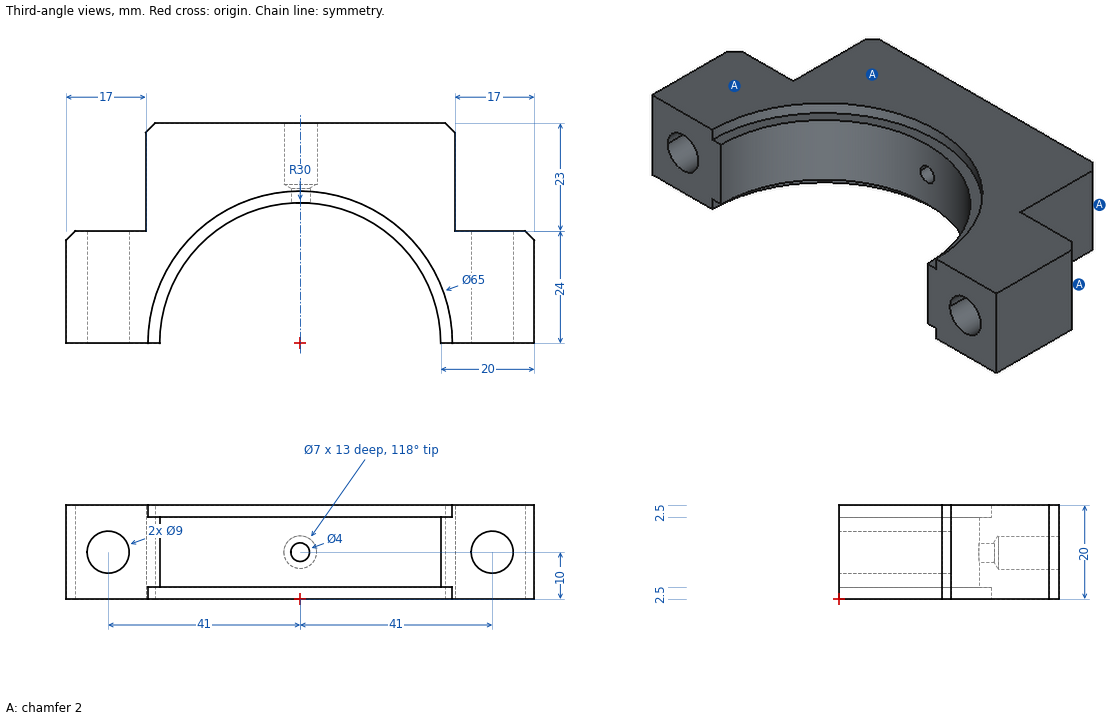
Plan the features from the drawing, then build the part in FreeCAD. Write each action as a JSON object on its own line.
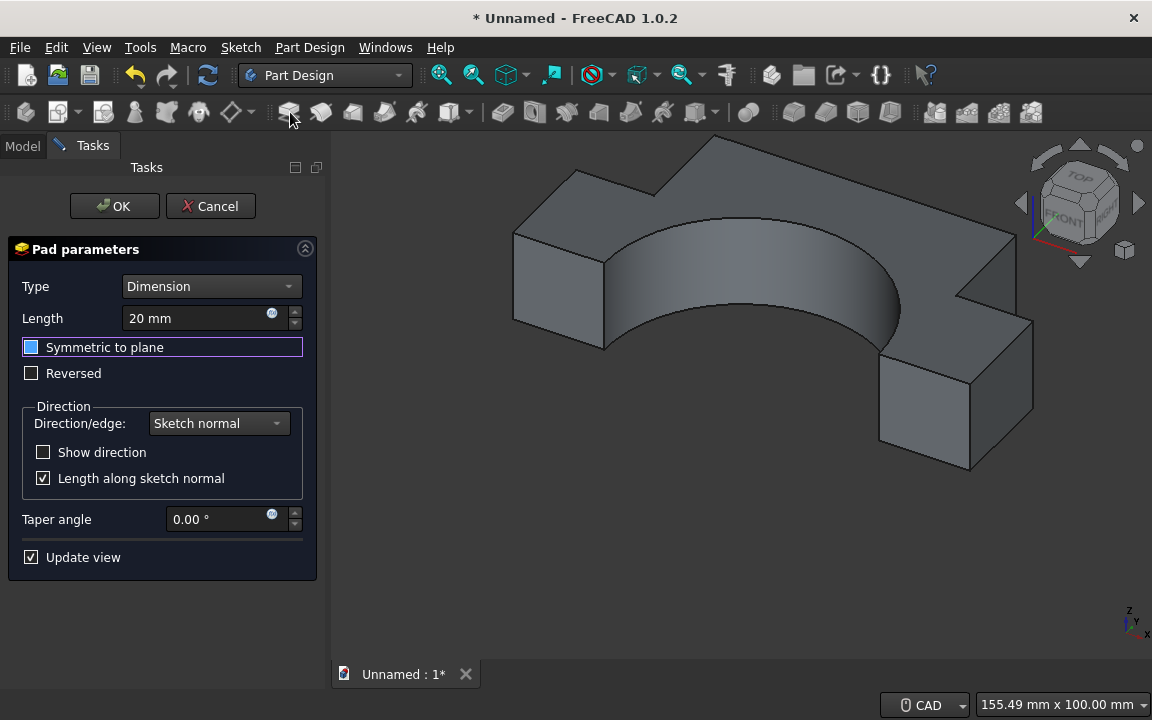
{"action": "left_click", "coordinate": [115, 206]}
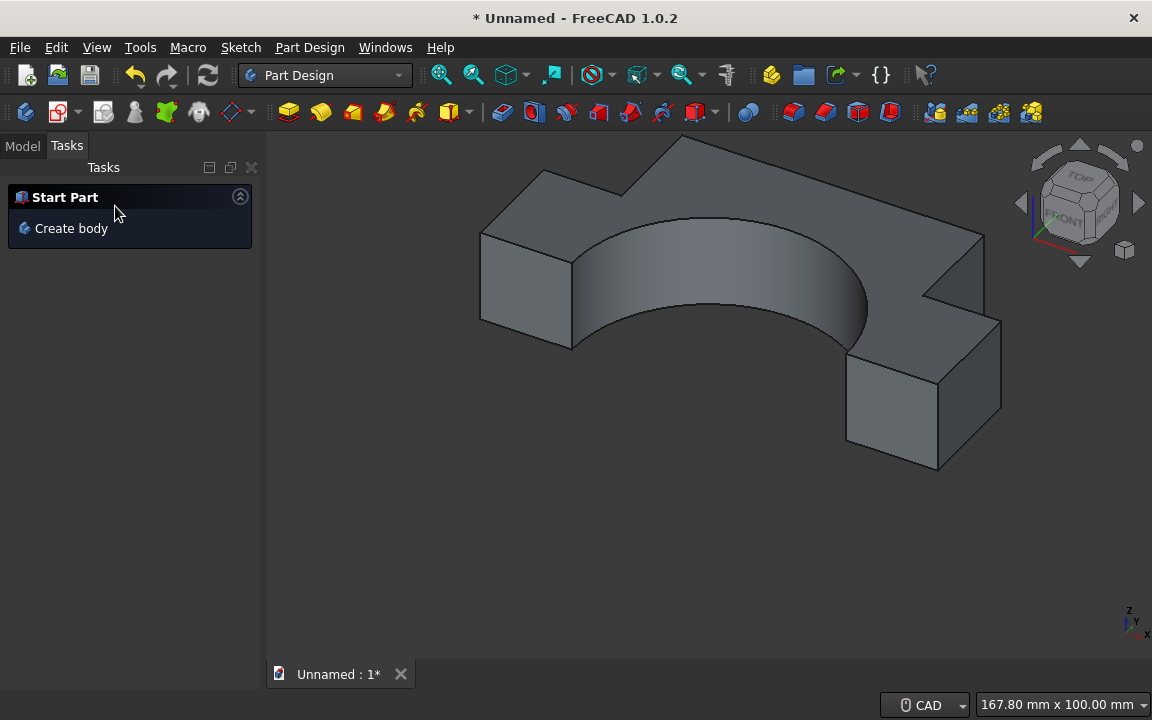
{"action": "left_click", "coordinate": [442, 76]}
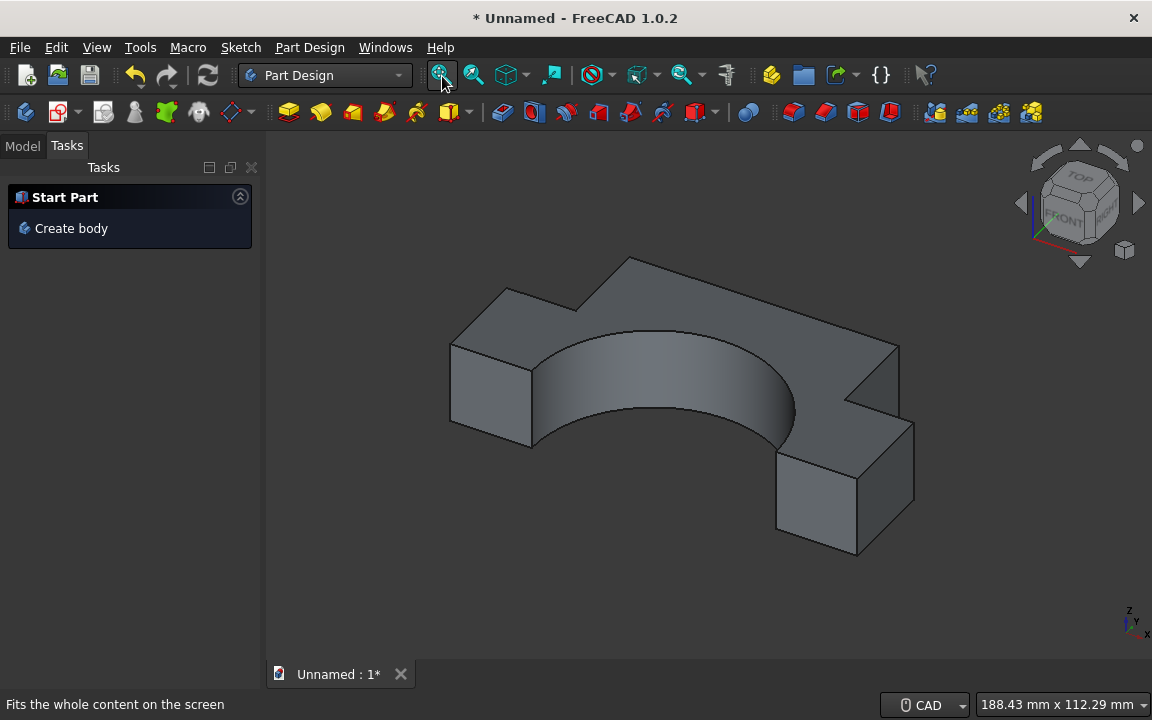
{"action": "key", "text": "0"}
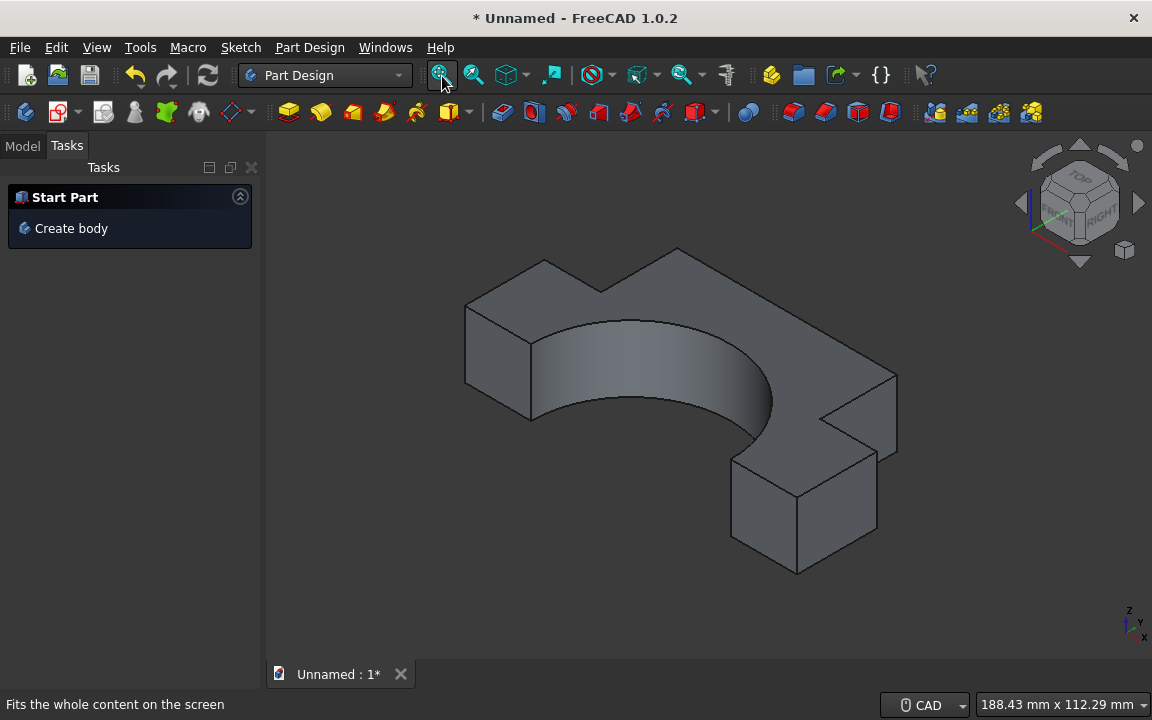
{"action": "key", "text": "2"}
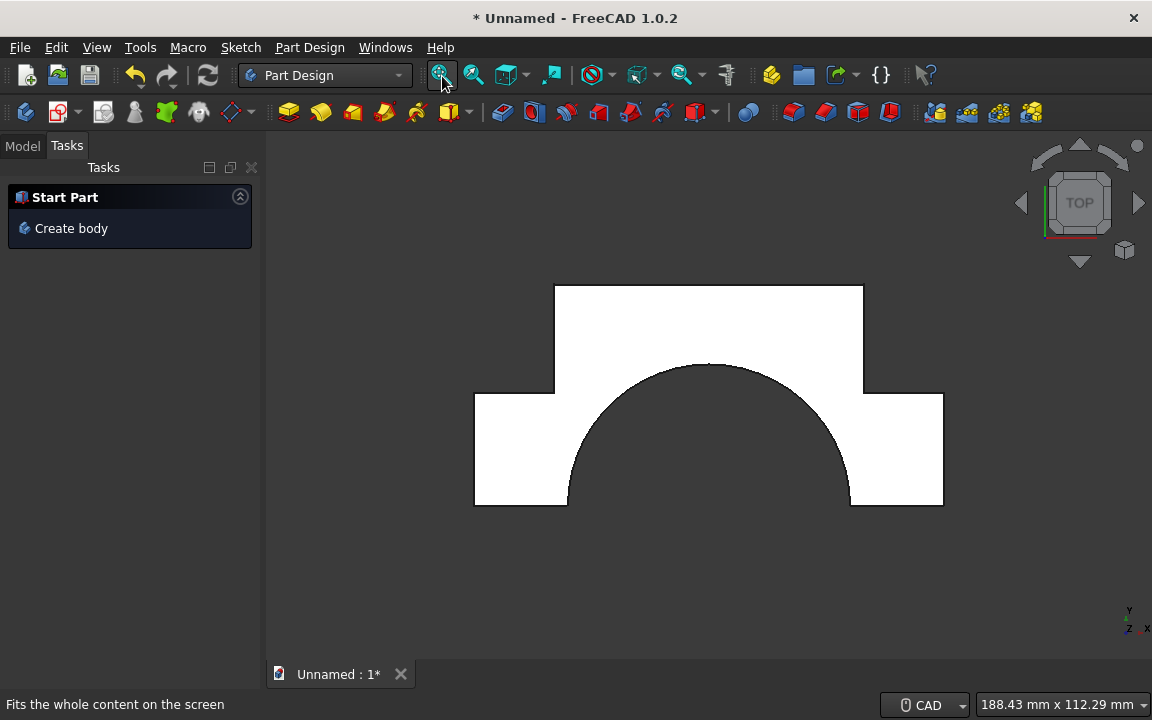
{"action": "key", "text": "1"}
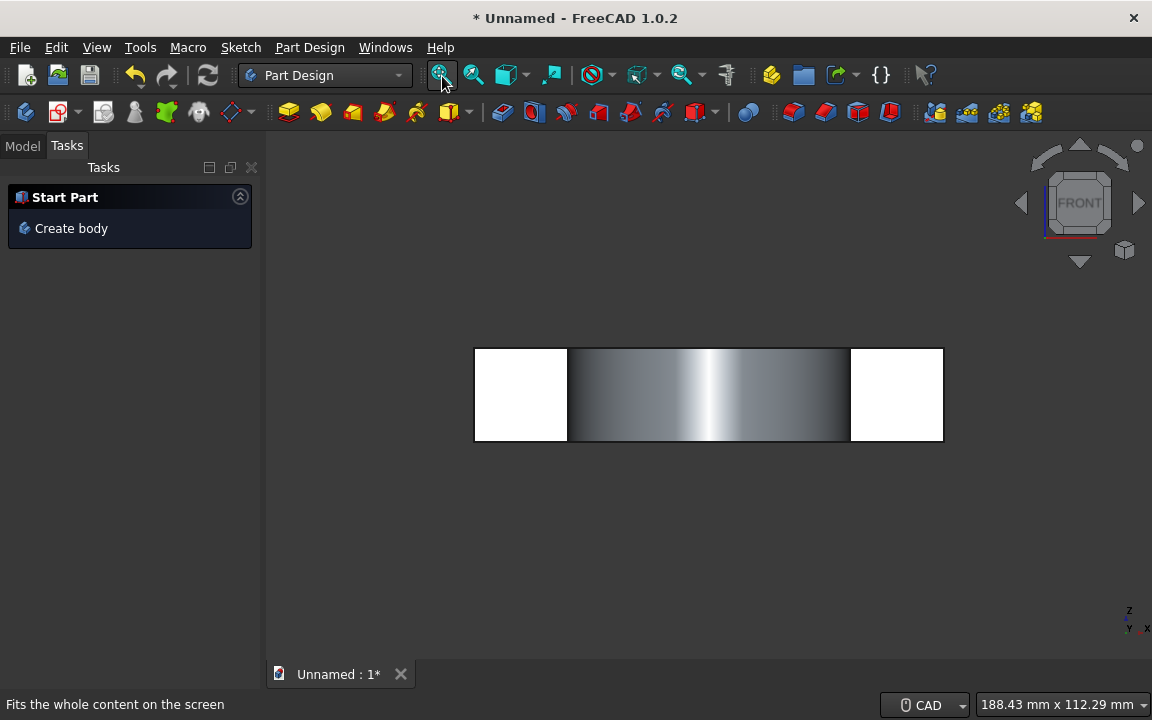
{"action": "key", "text": "3"}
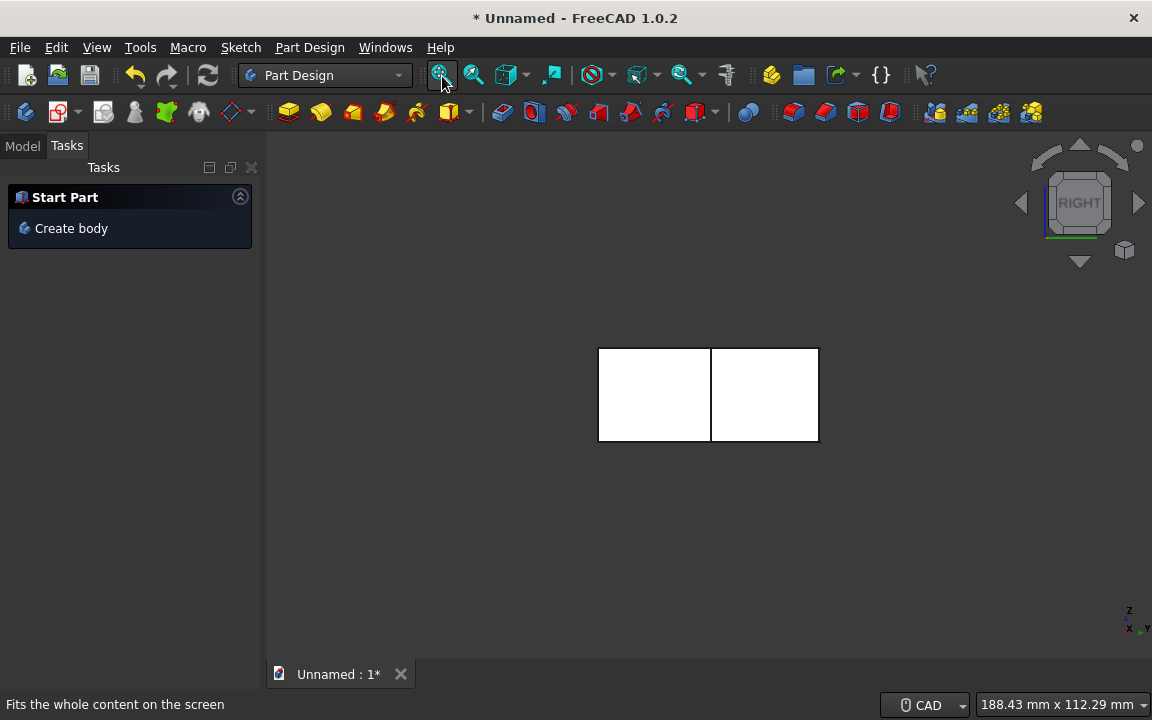
{"action": "left_click", "coordinate": [442, 76]}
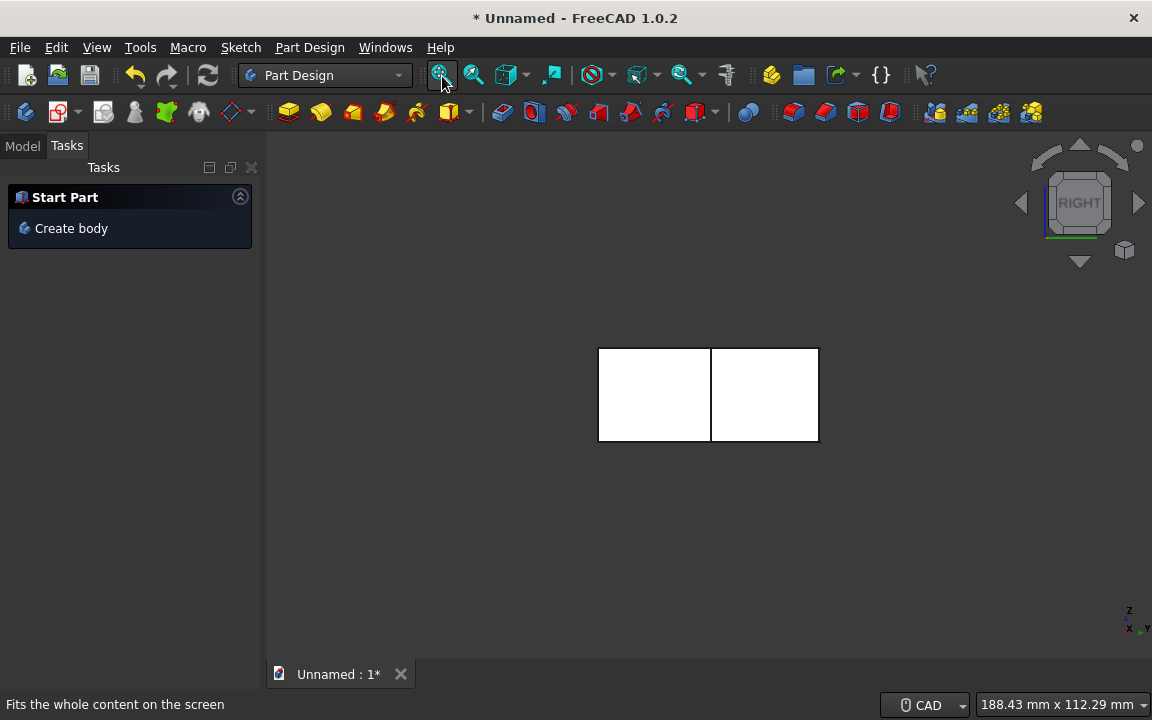
{"action": "left_click", "coordinate": [819, 394]}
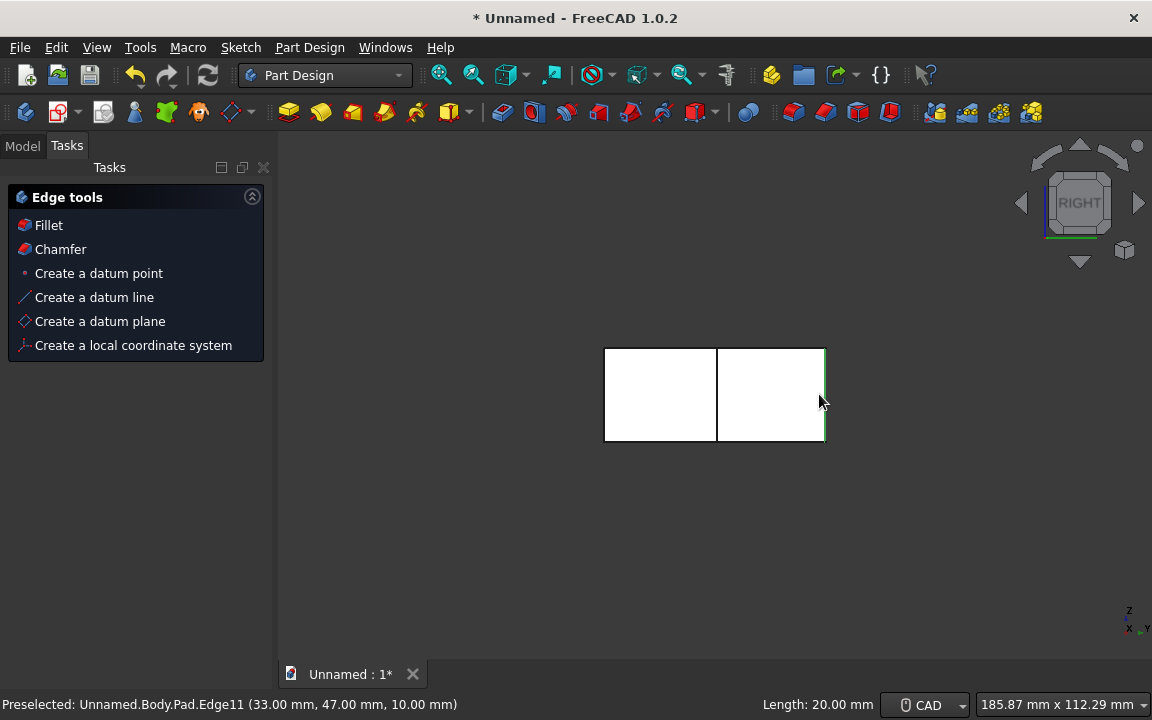
{"action": "left_click", "coordinate": [717, 394], "text": "ctrl"}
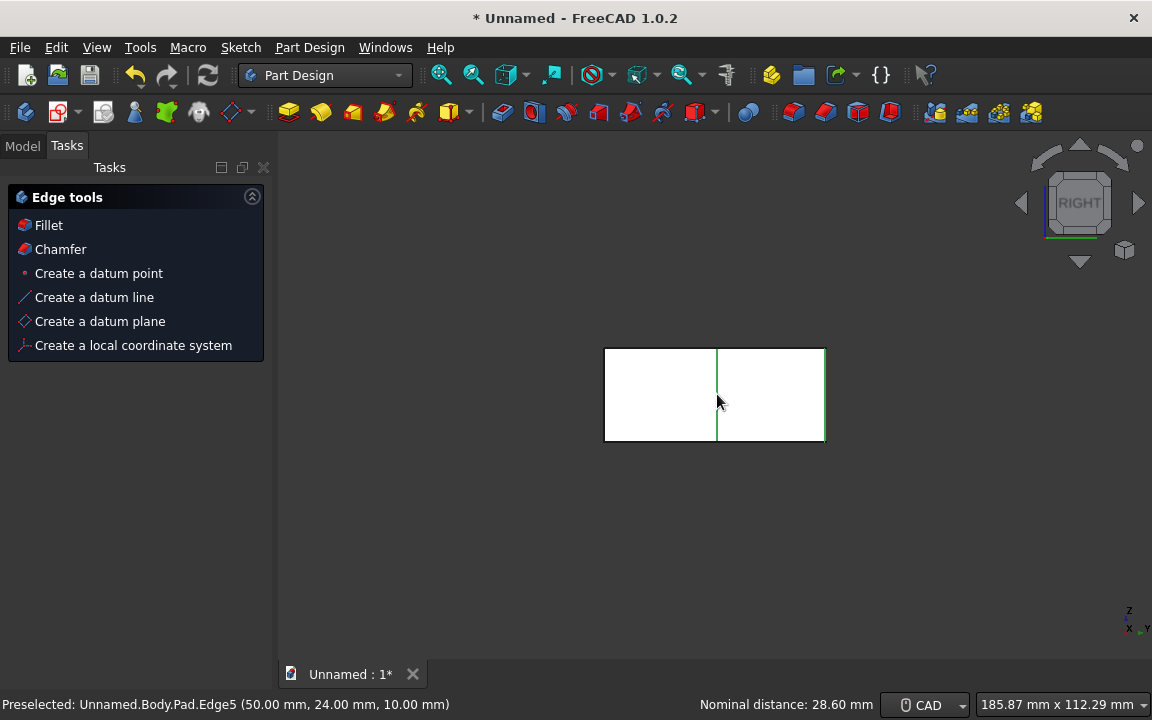
{"action": "key", "text": "5"}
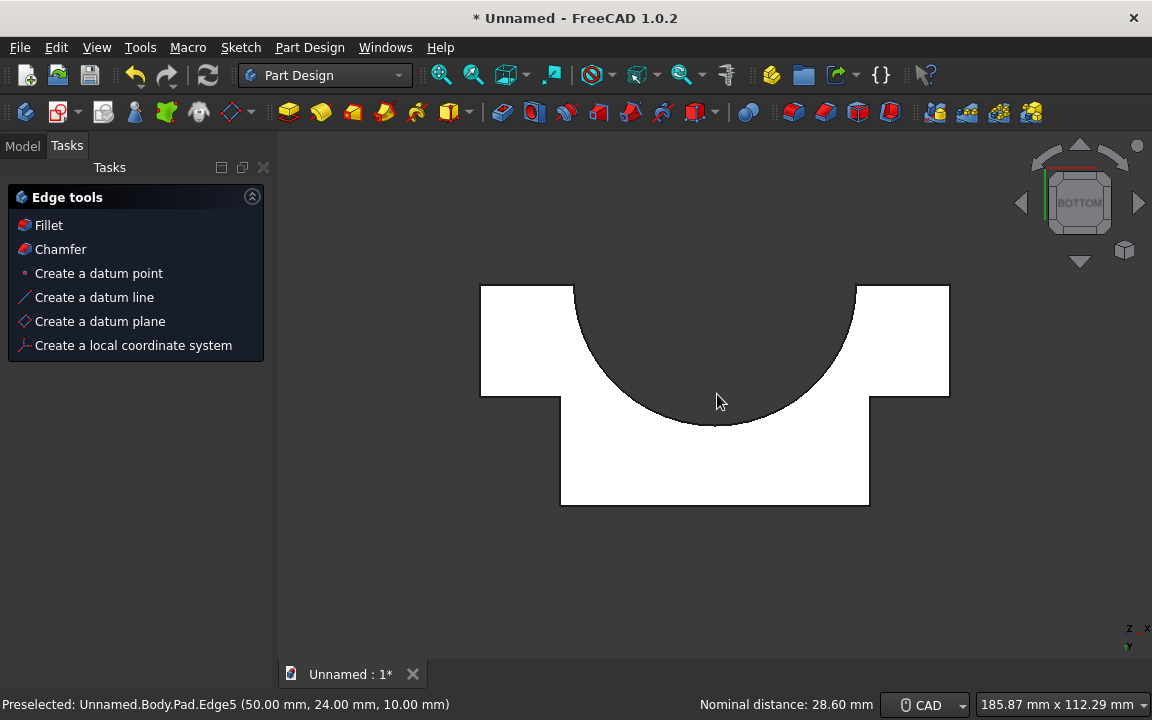
{"action": "key", "text": "4"}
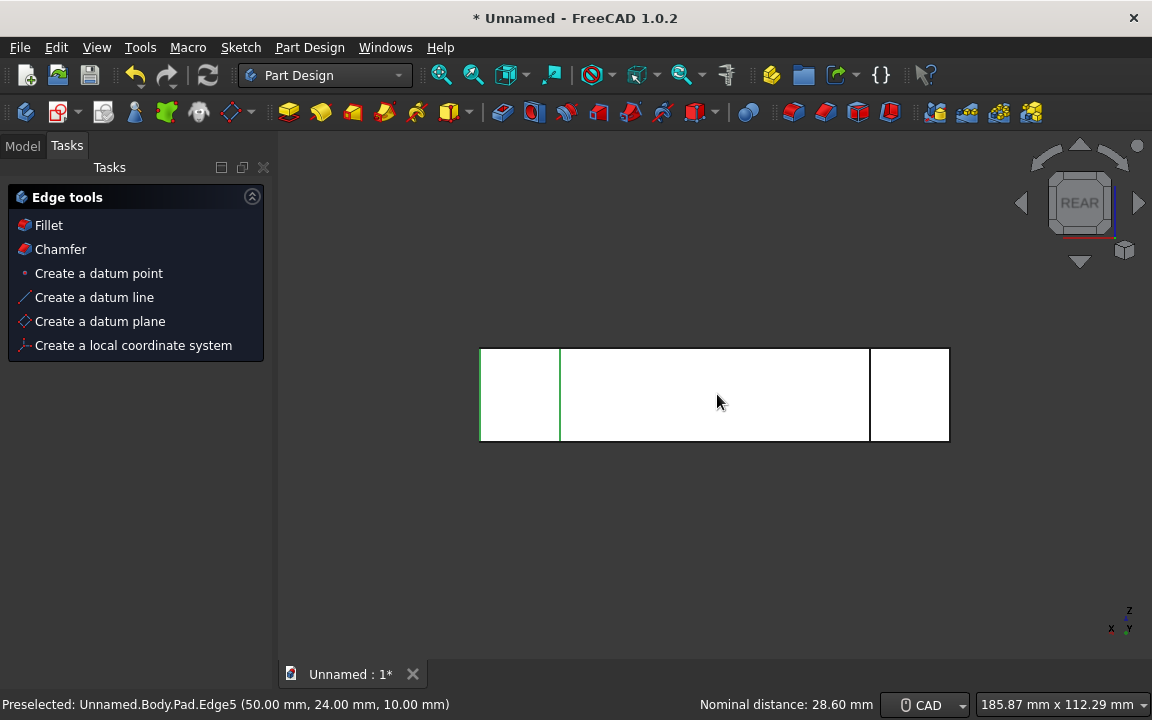
{"action": "left_click", "coordinate": [950, 394], "text": "ctrl"}